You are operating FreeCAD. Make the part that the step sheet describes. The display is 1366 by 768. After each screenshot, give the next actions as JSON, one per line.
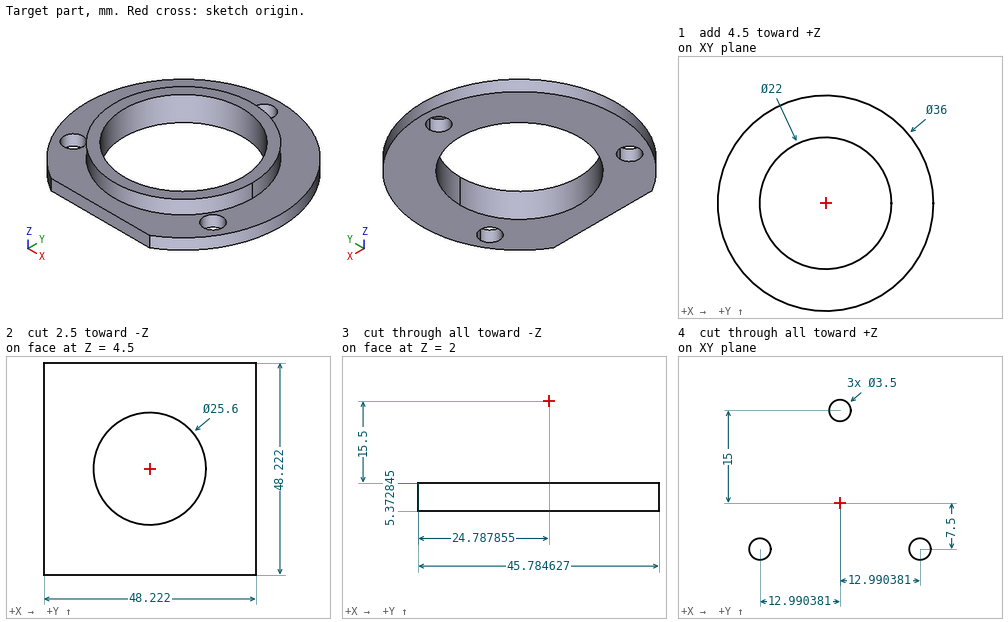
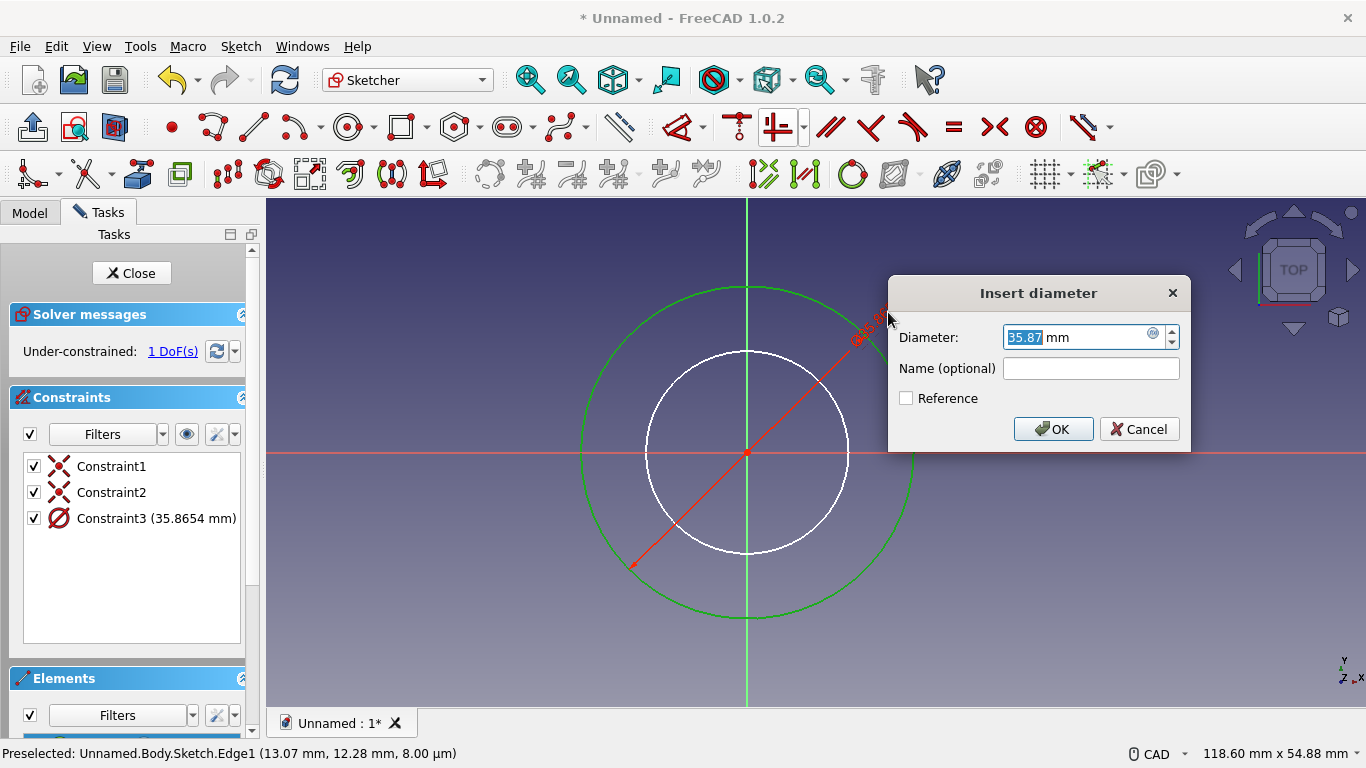
{"action": "type", "text": "36"}
{"action": "key", "text": "Return"}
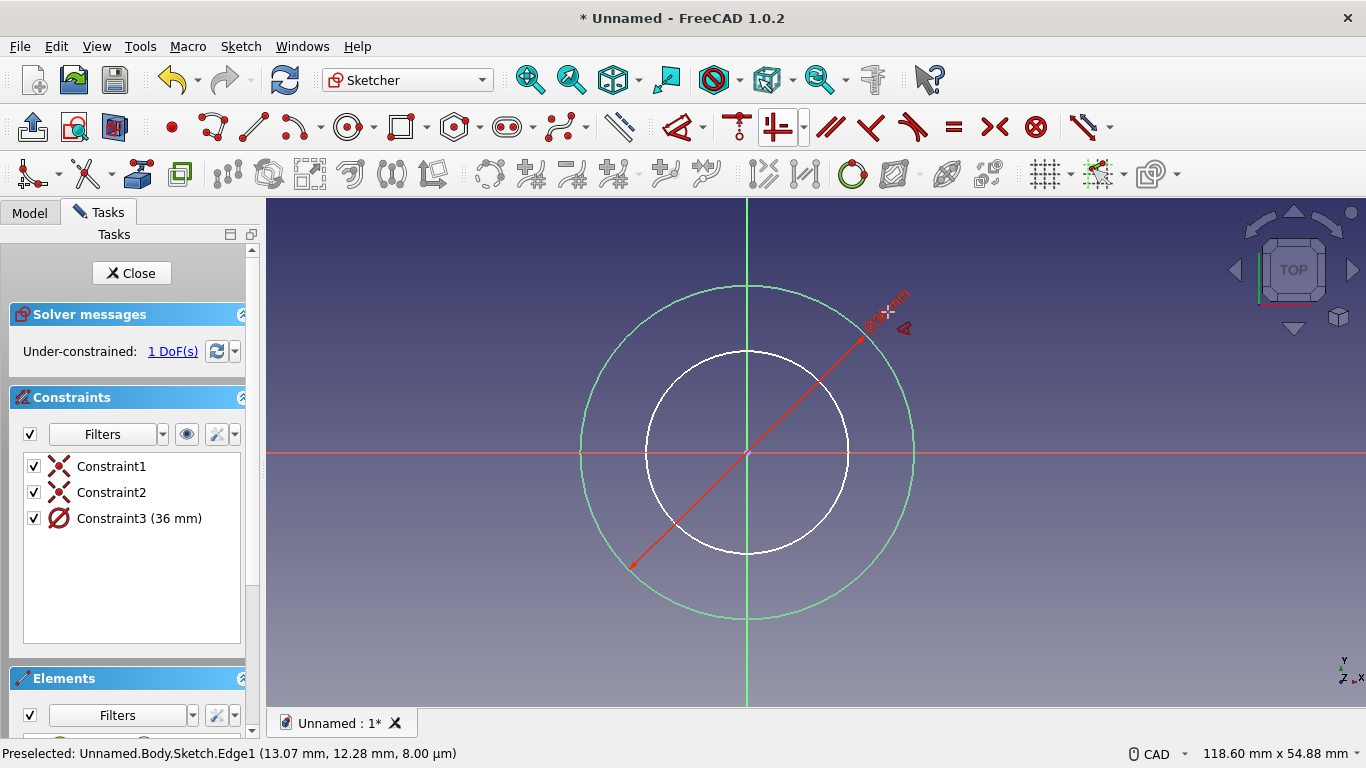
{"action": "left_click", "coordinate": [819, 381]}
{"action": "left_click", "coordinate": [842, 358]}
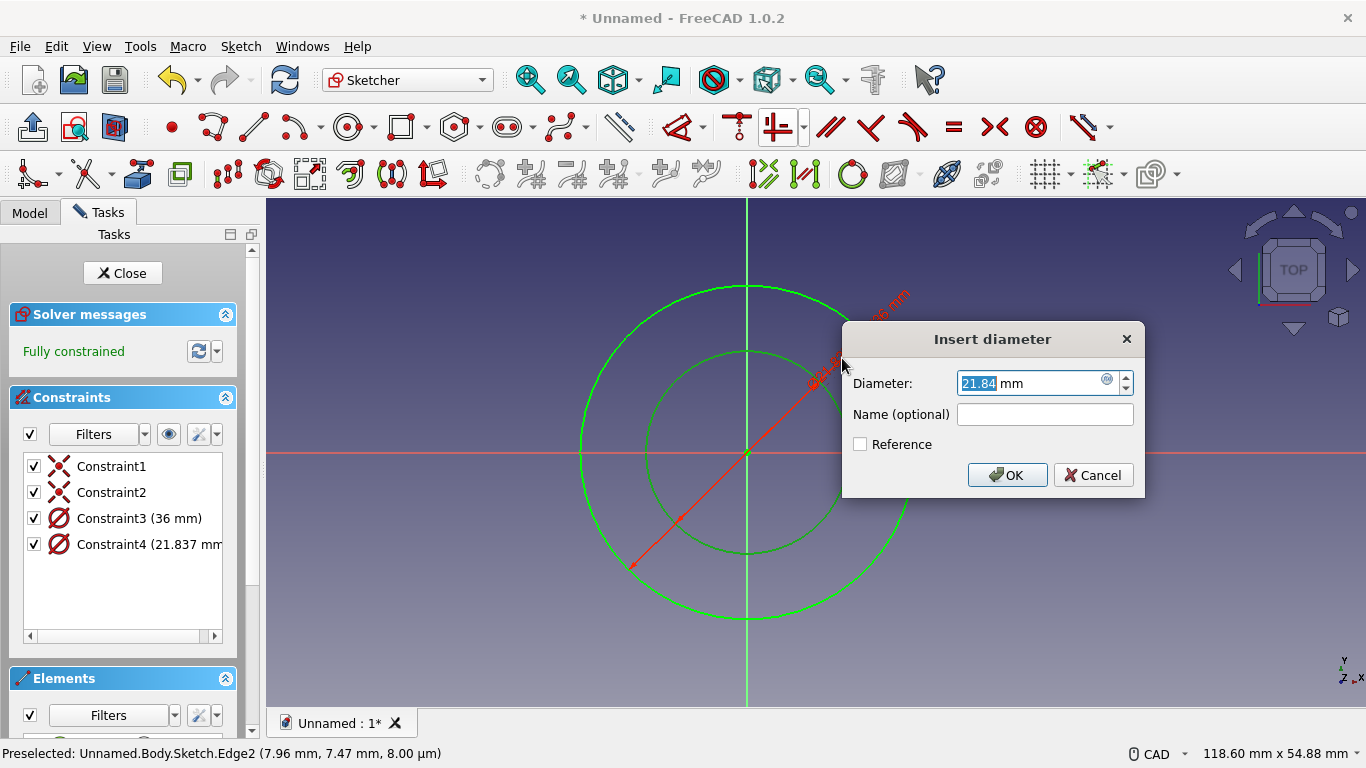
{"action": "type", "text": "22"}
{"action": "key", "text": "Return"}
{"action": "key", "text": "Escape"}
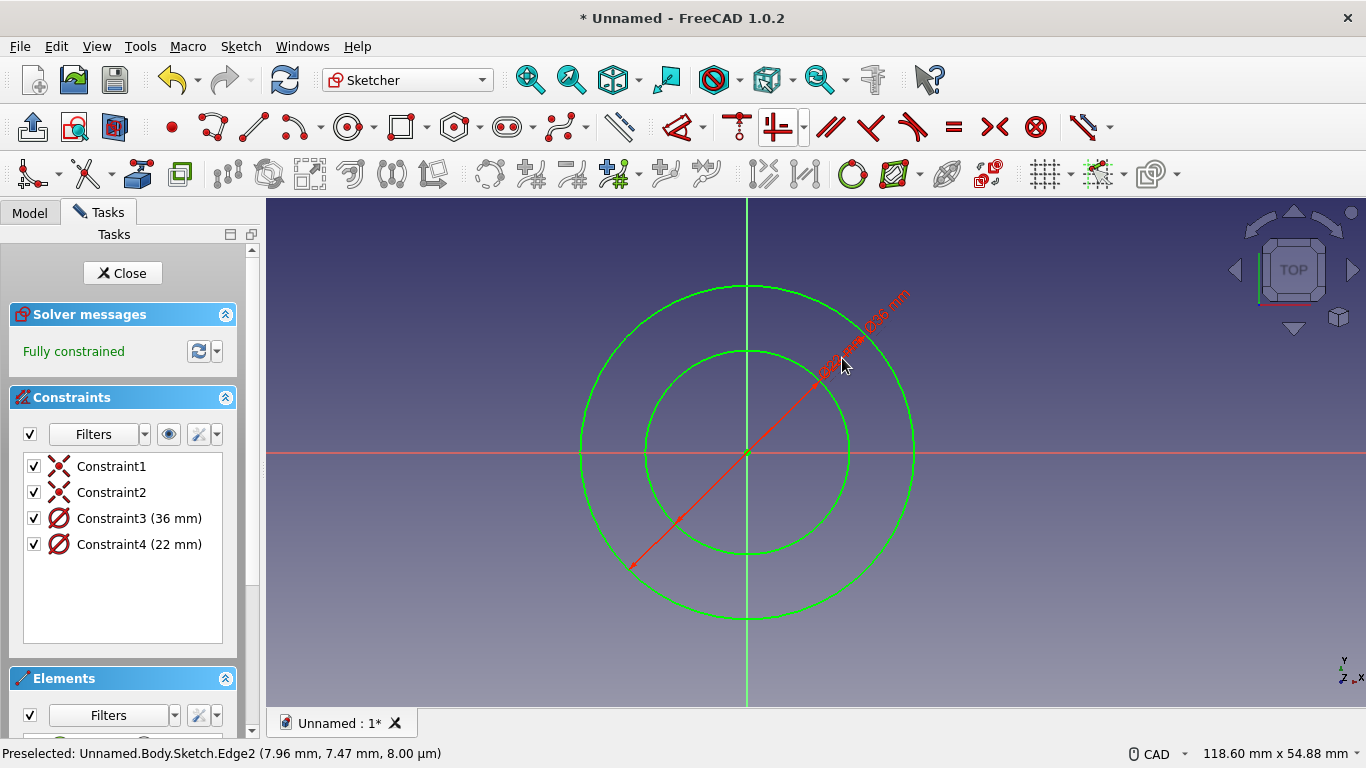
{"action": "left_click", "coordinate": [123, 273]}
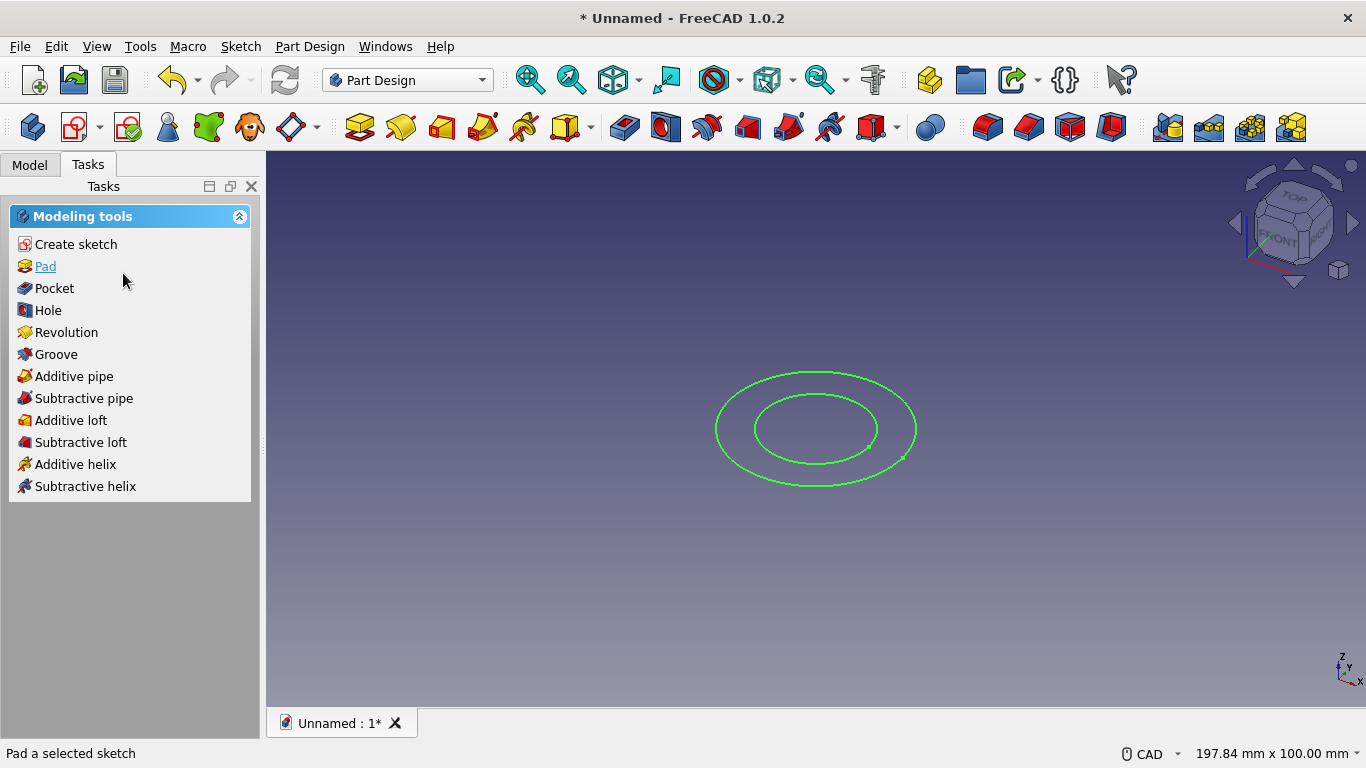
{"action": "left_click", "coordinate": [360, 128]}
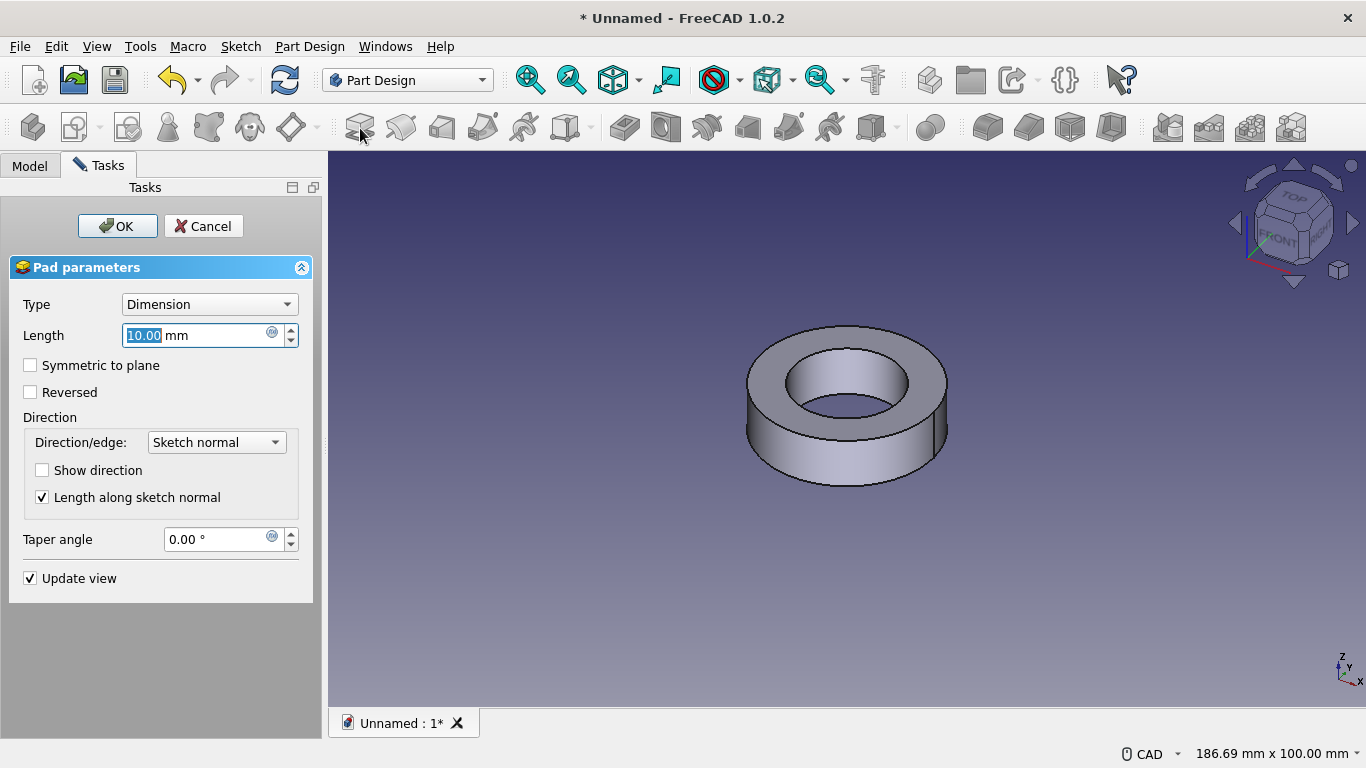
{"action": "type", "text": "4.5"}
{"action": "key", "text": "Tab"}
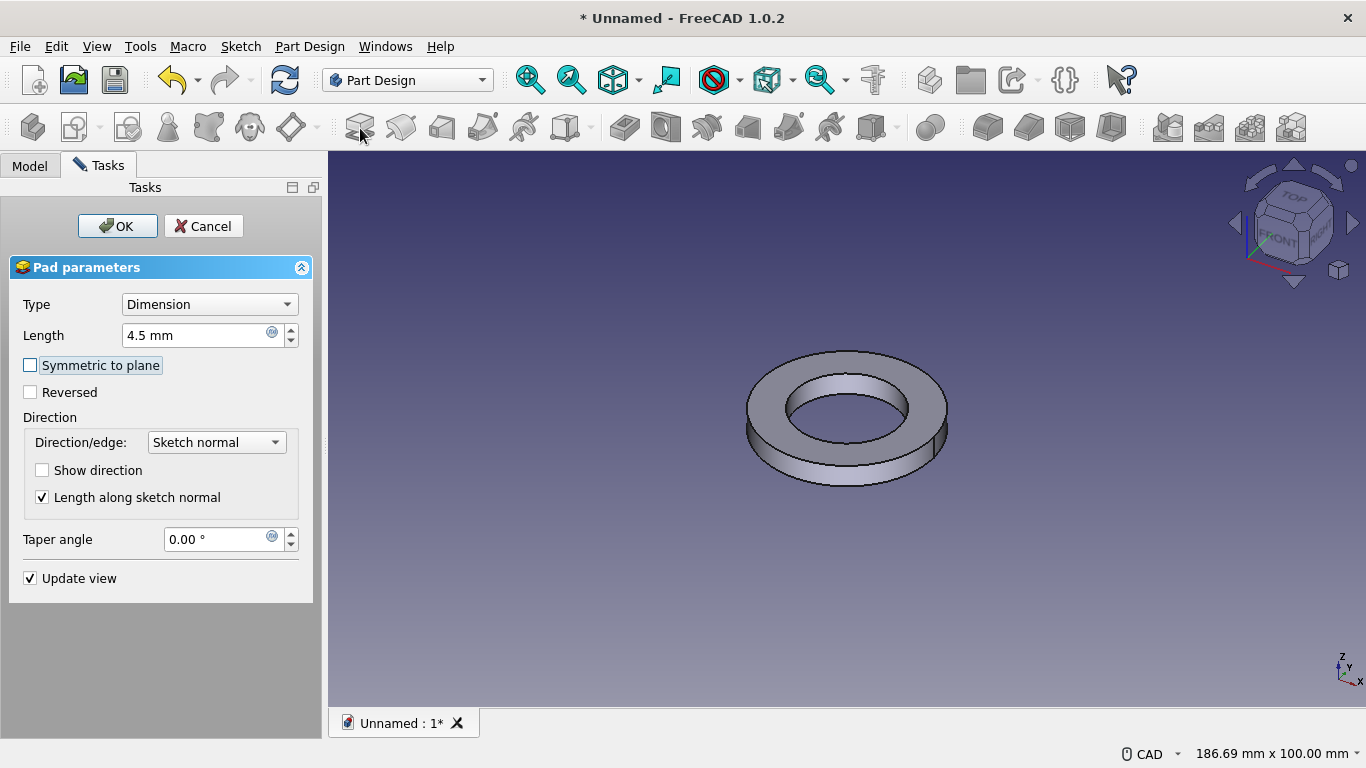
{"action": "left_click", "coordinate": [118, 226]}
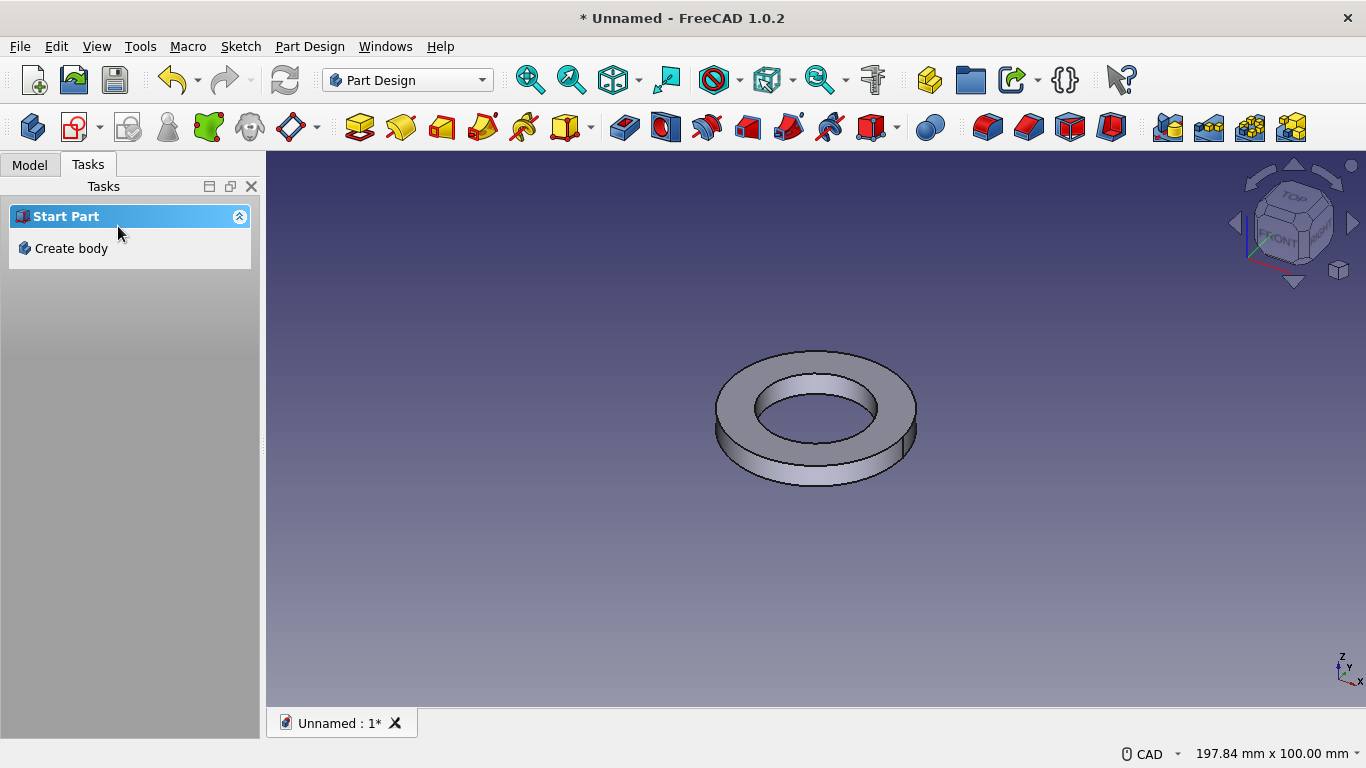
{"action": "left_click", "coordinate": [531, 80]}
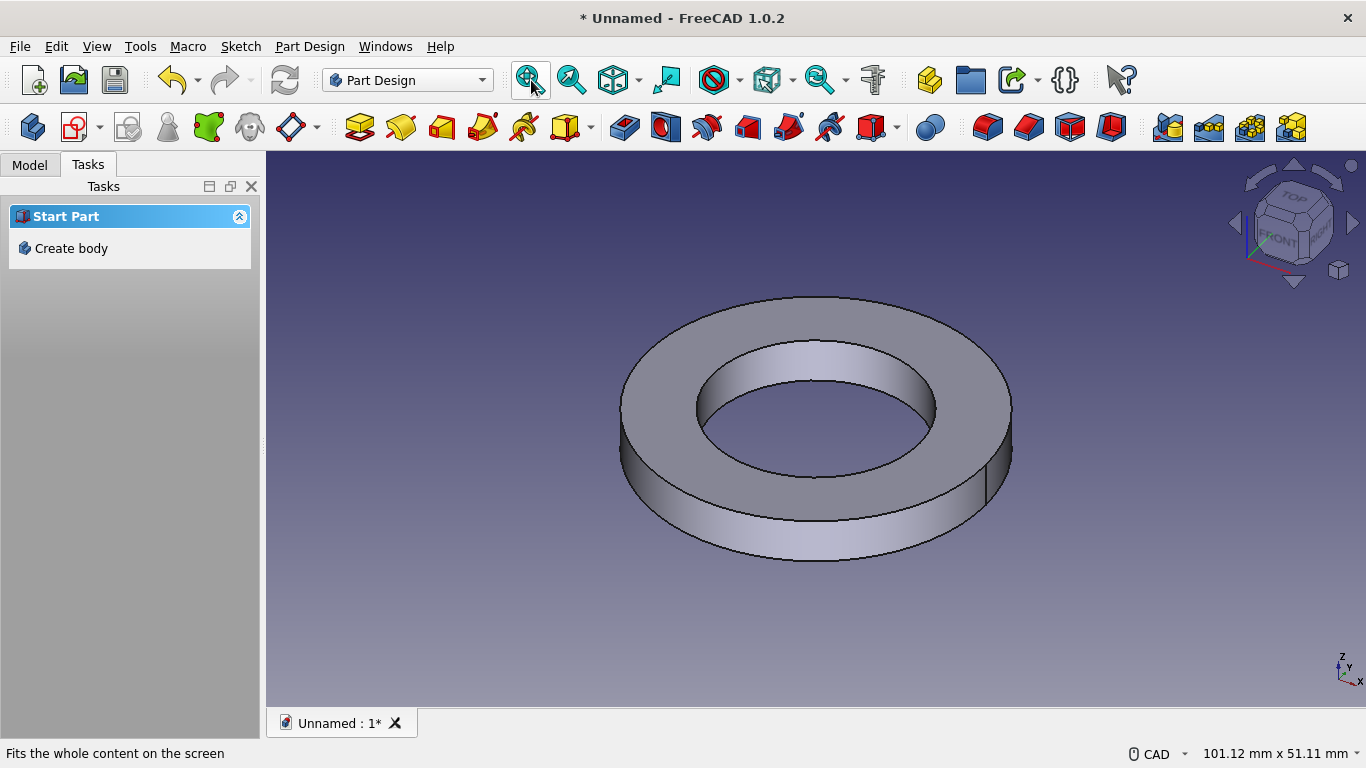
{"action": "left_click", "coordinate": [663, 431]}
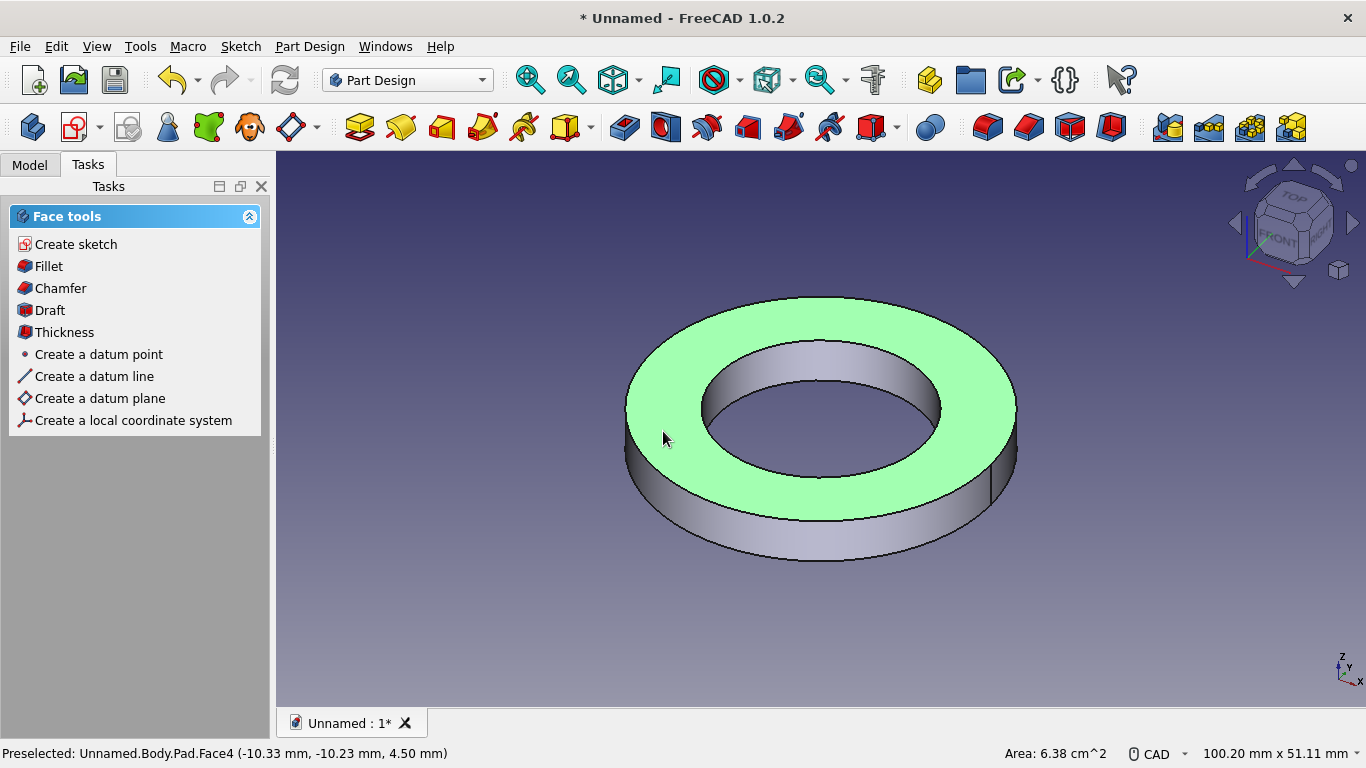
{"action": "left_click", "coordinate": [74, 128]}